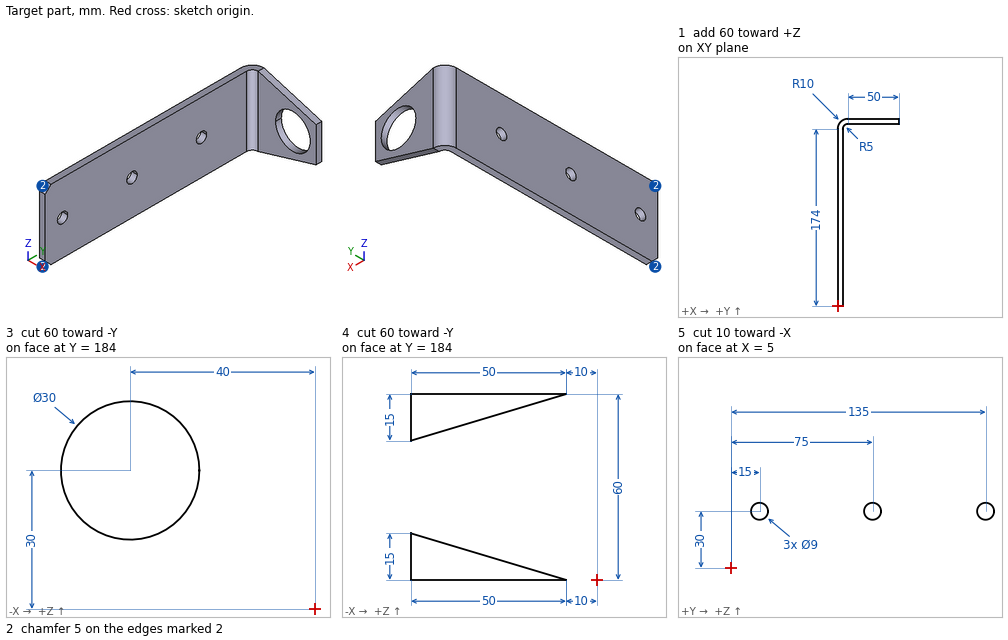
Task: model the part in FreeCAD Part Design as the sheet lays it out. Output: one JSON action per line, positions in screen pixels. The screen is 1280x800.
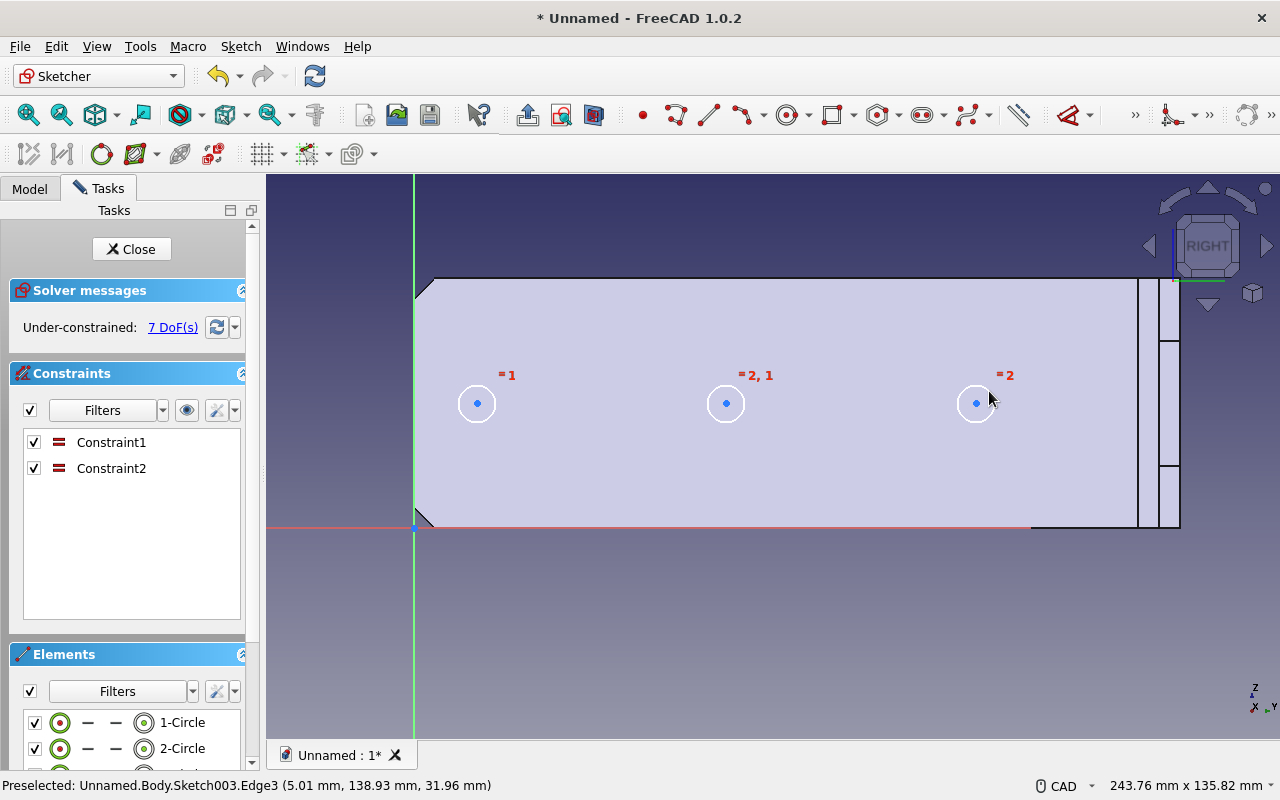
{"action": "left_click", "coordinate": [477, 404]}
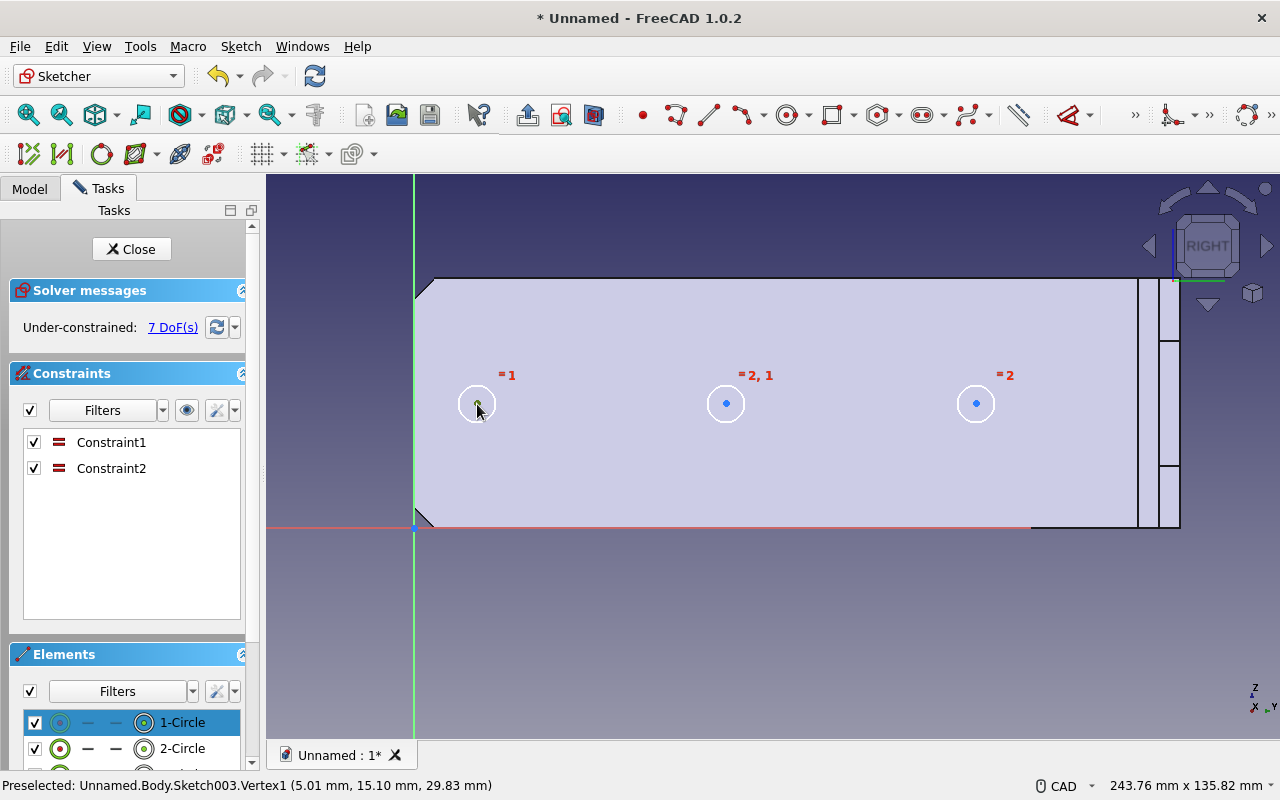
{"action": "left_click", "coordinate": [726, 404]}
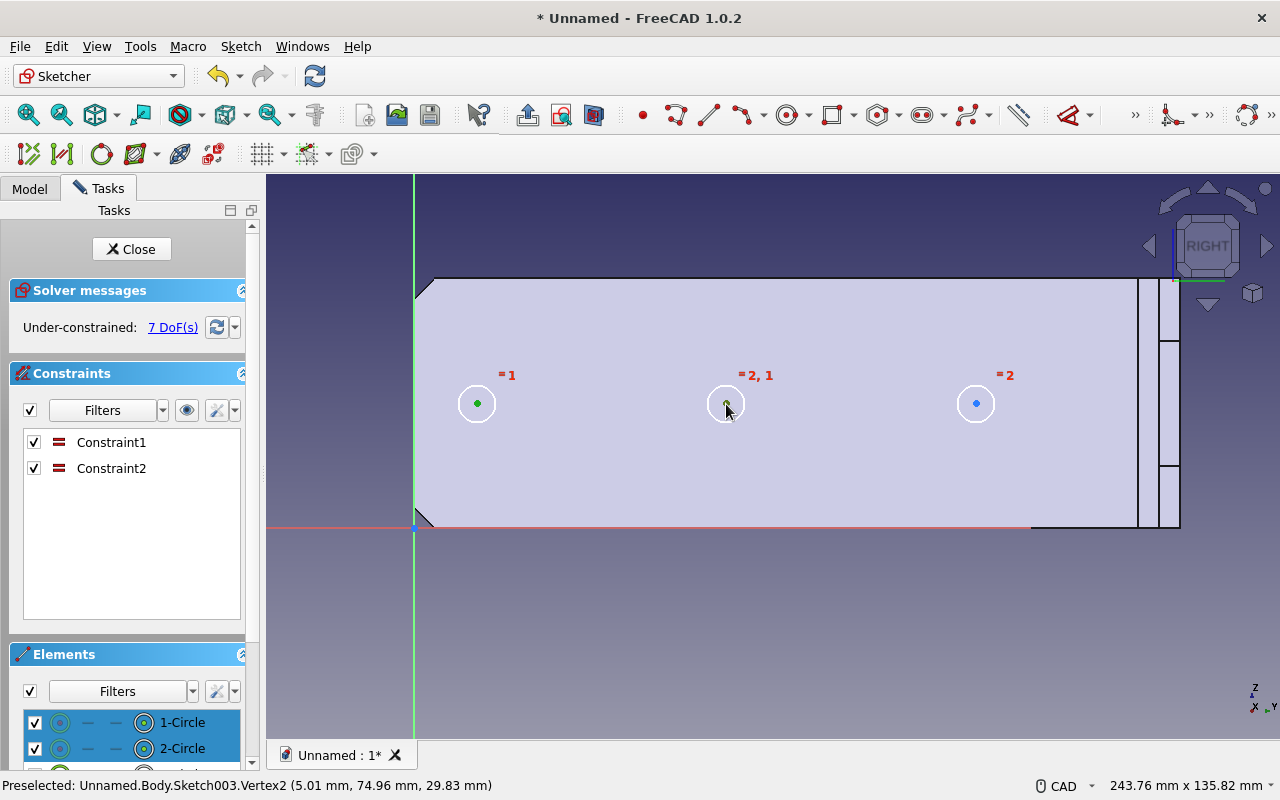
{"action": "key", "text": "h"}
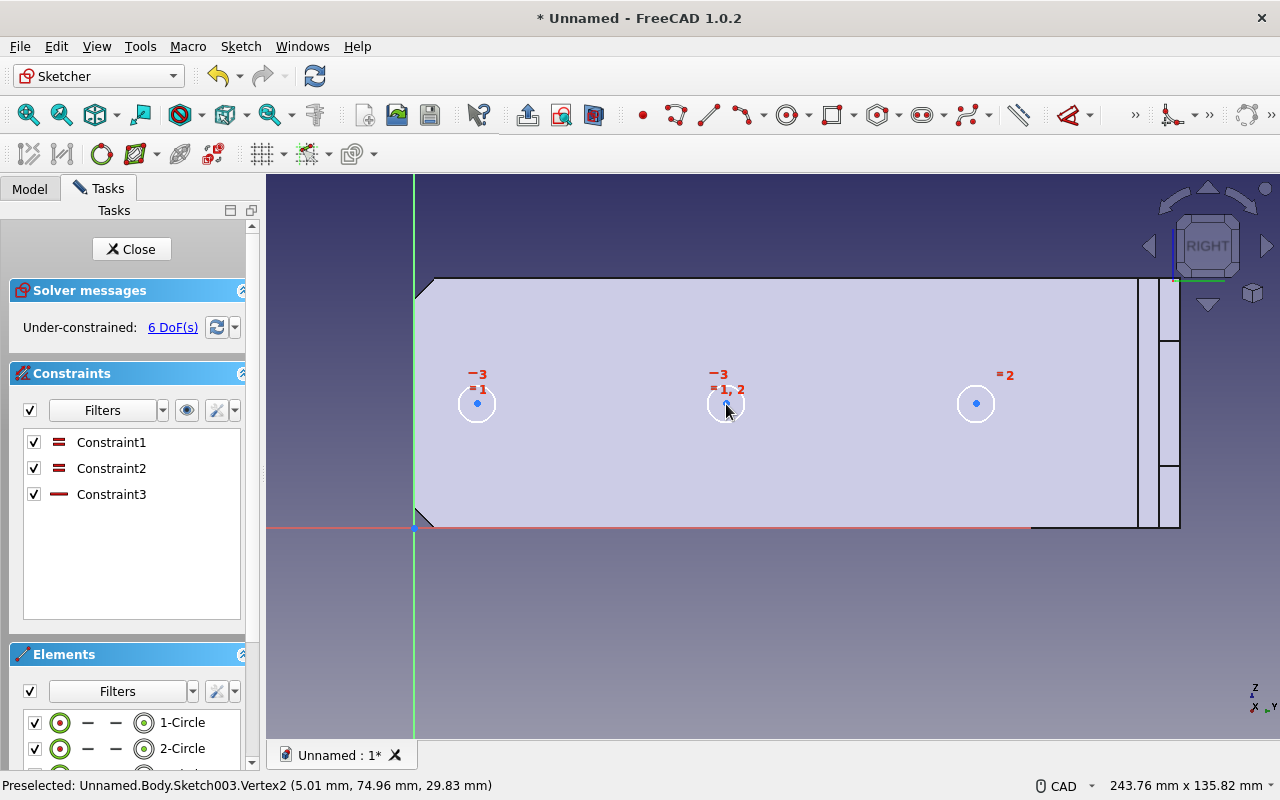
{"action": "left_click", "coordinate": [726, 404]}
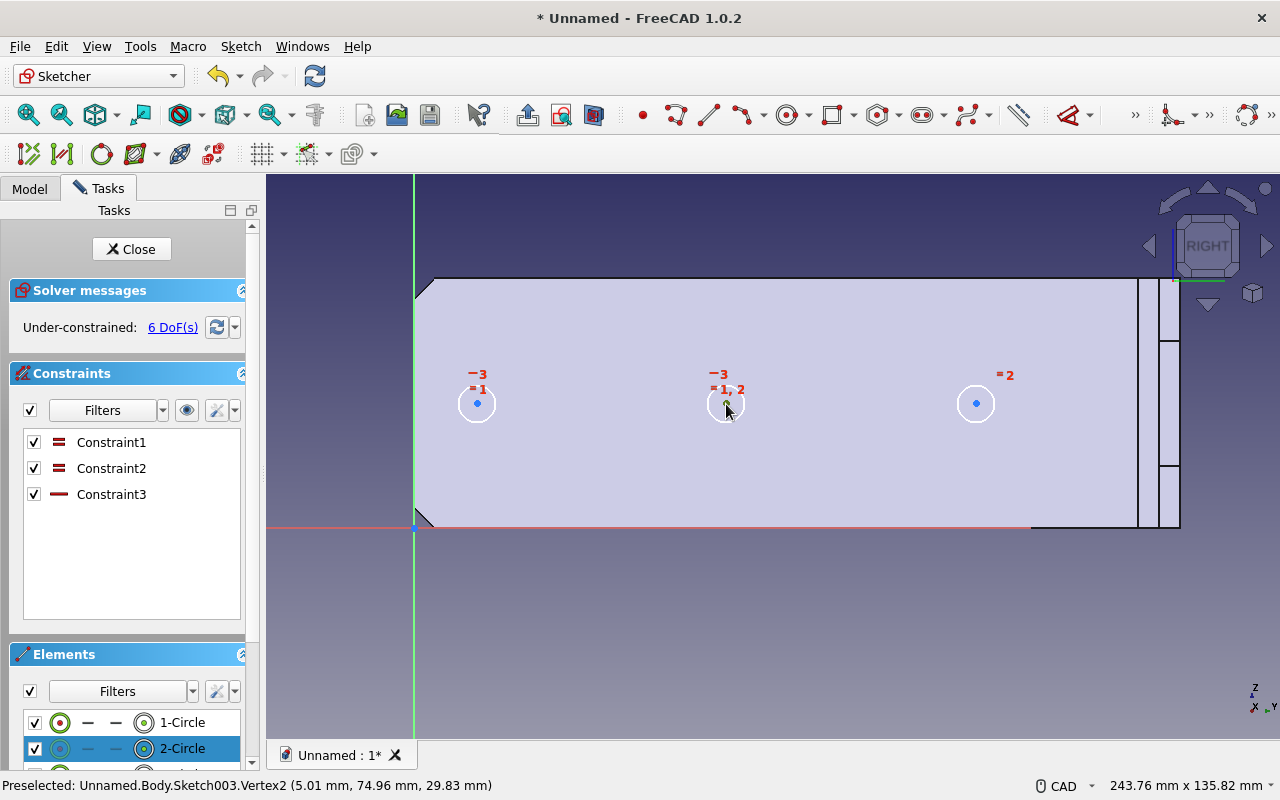
{"action": "left_click", "coordinate": [976, 404]}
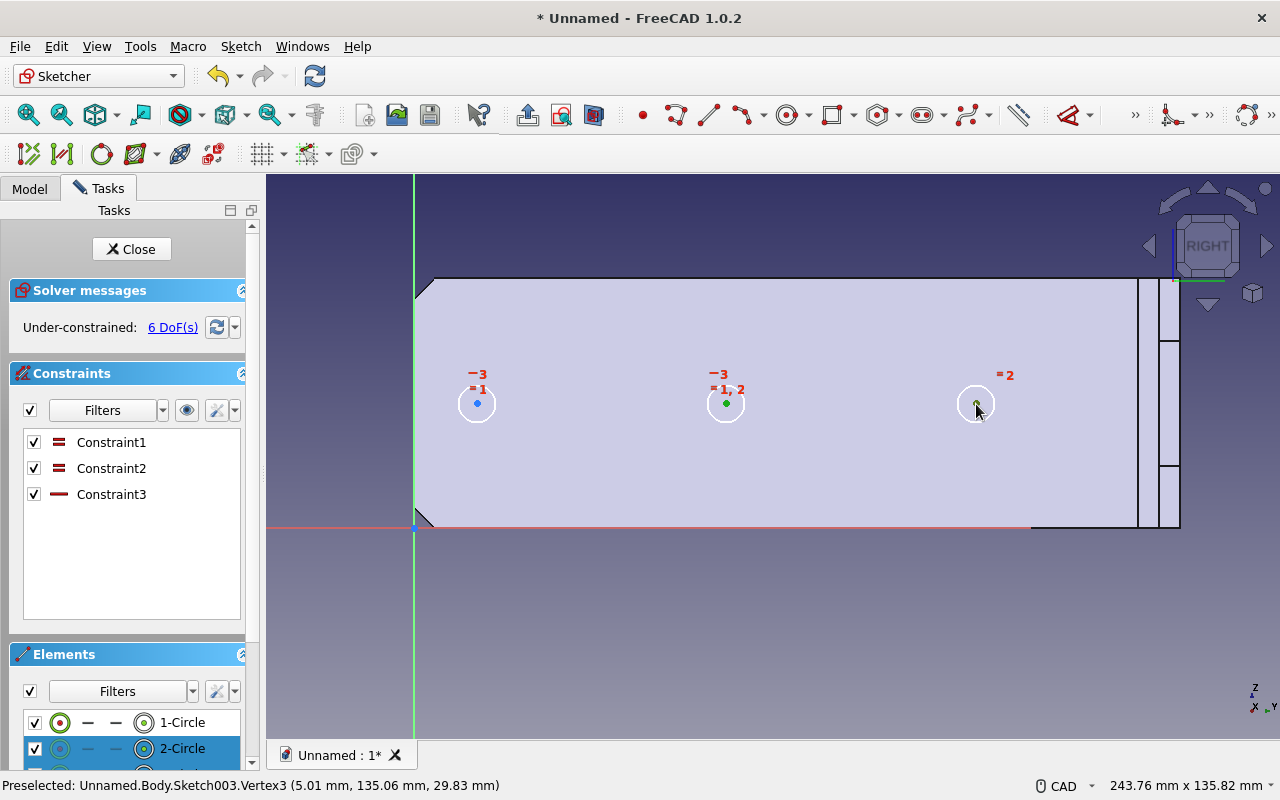
{"action": "key", "text": "h"}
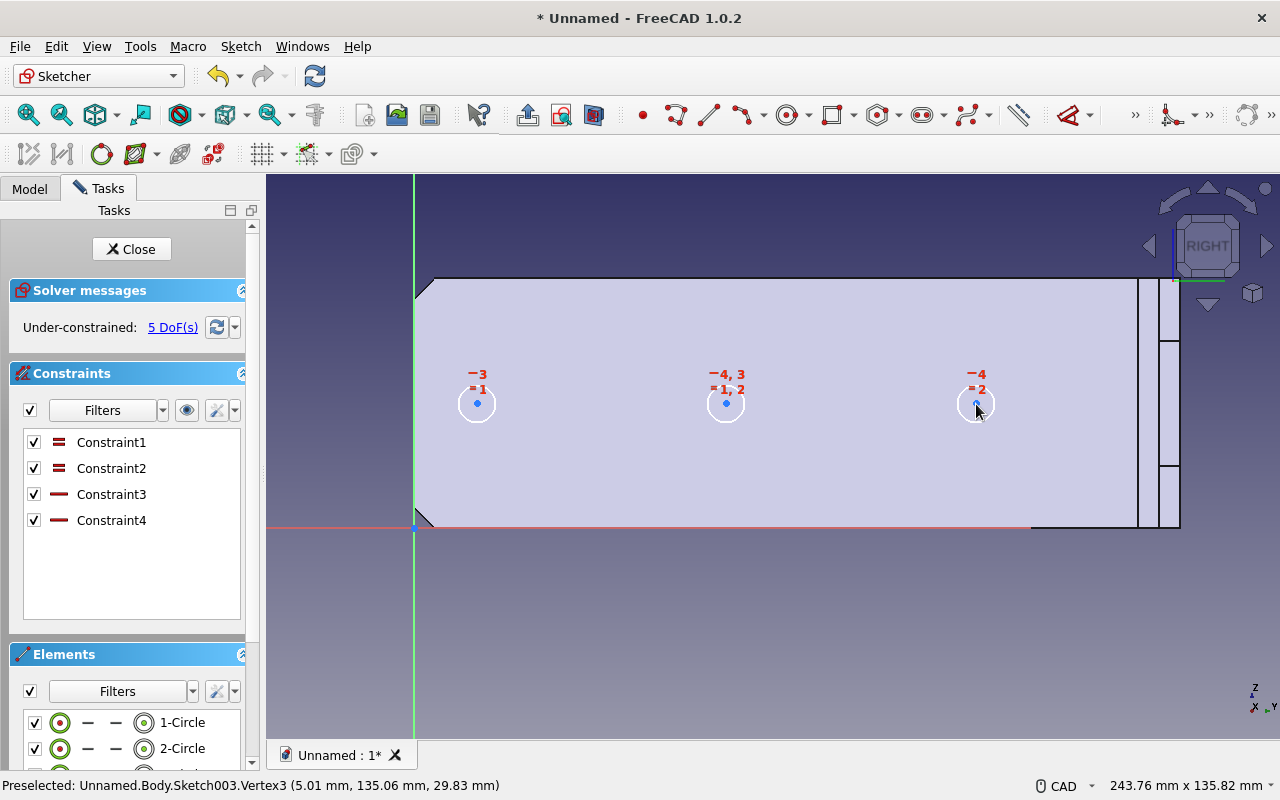
{"action": "key", "text": "d"}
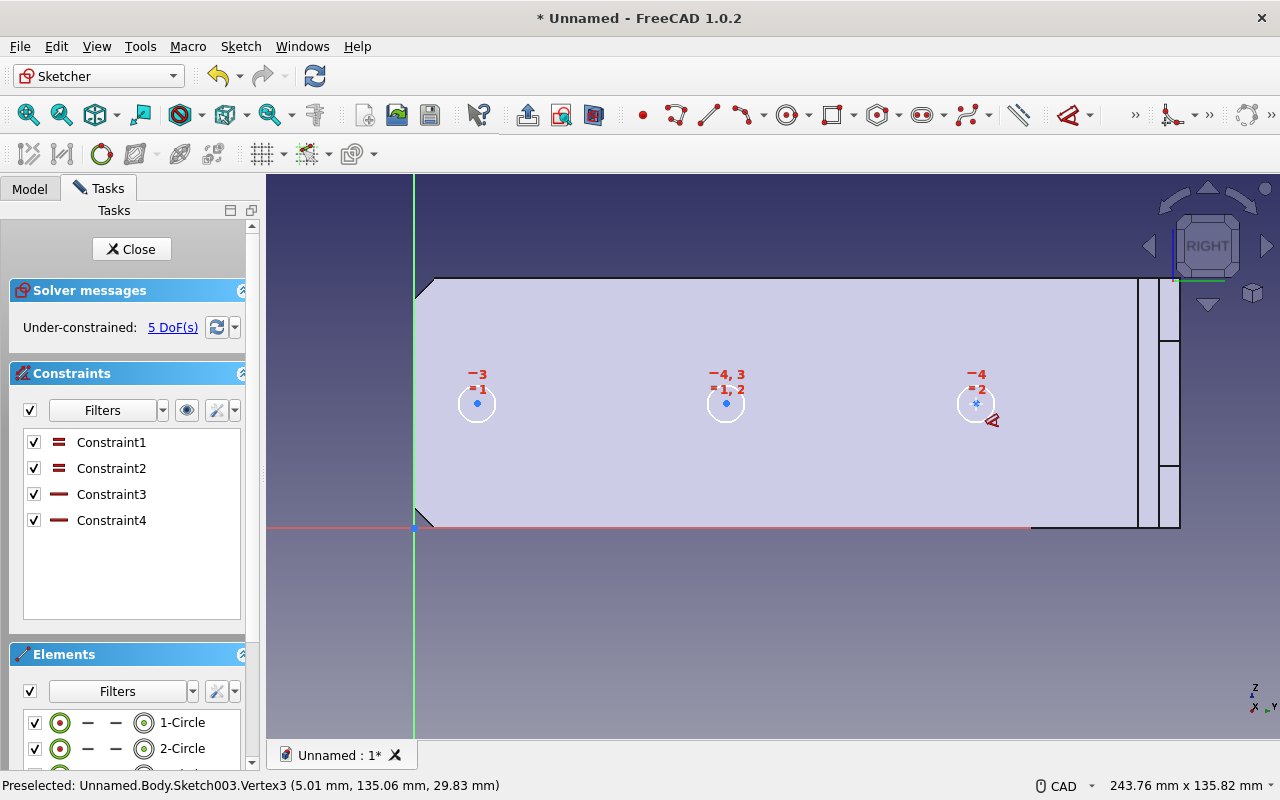
{"action": "left_click", "coordinate": [490, 391]}
{"action": "left_click", "coordinate": [513, 368]}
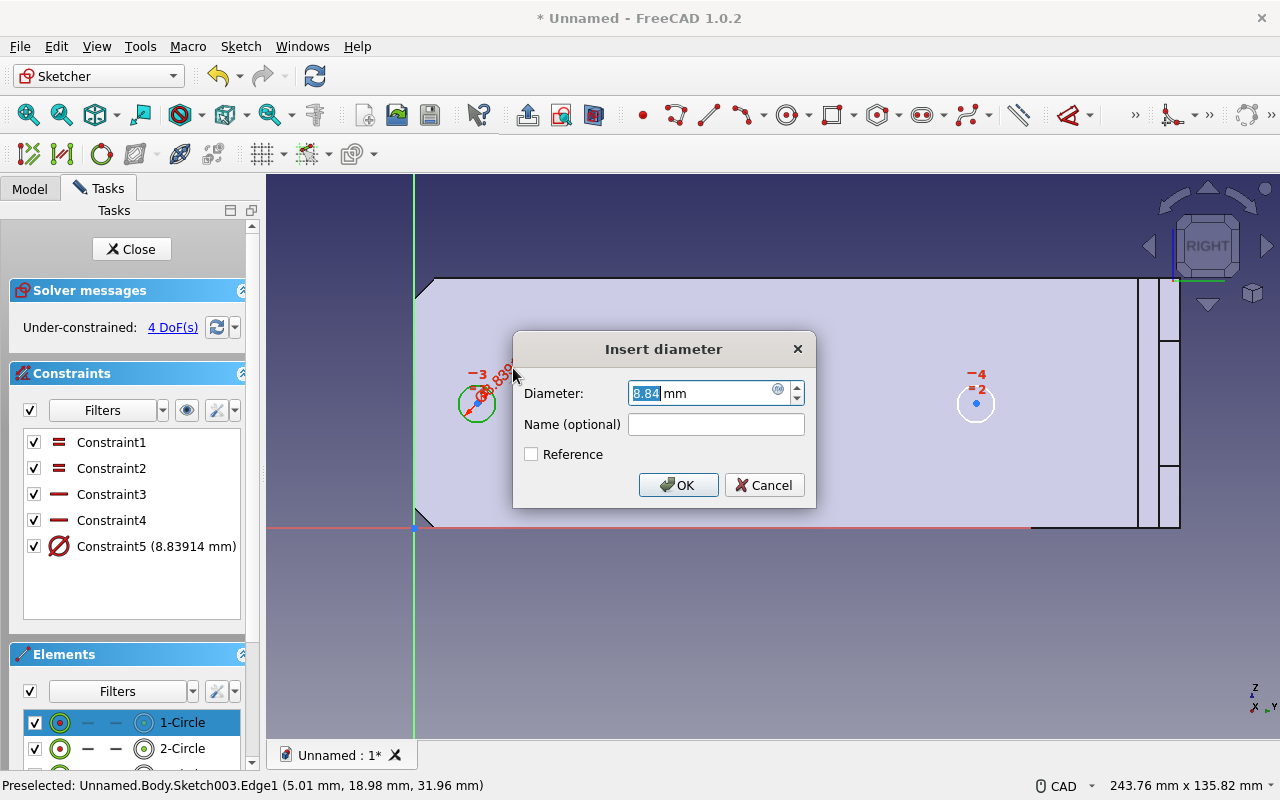
{"action": "type", "text": "9"}
{"action": "key", "text": "Return"}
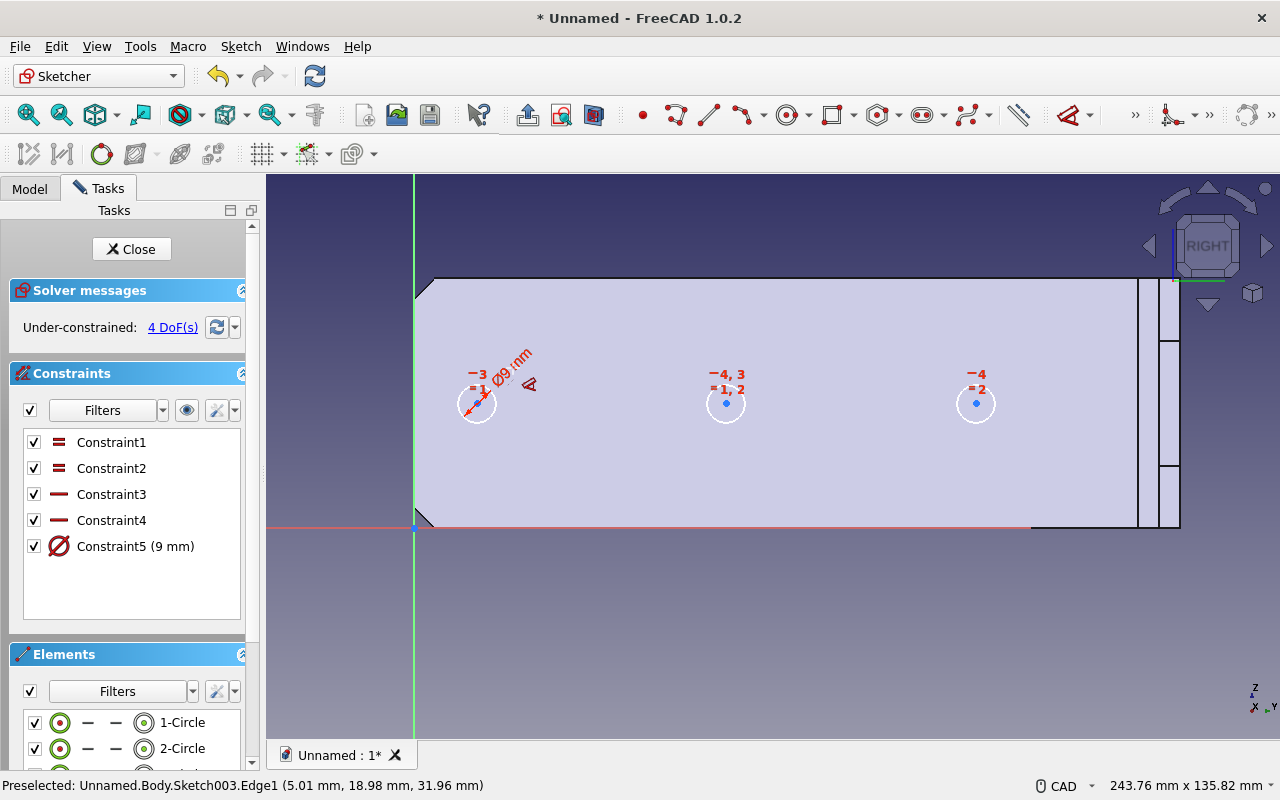
{"action": "left_click", "coordinate": [477, 404]}
{"action": "left_click", "coordinate": [446, 562]}